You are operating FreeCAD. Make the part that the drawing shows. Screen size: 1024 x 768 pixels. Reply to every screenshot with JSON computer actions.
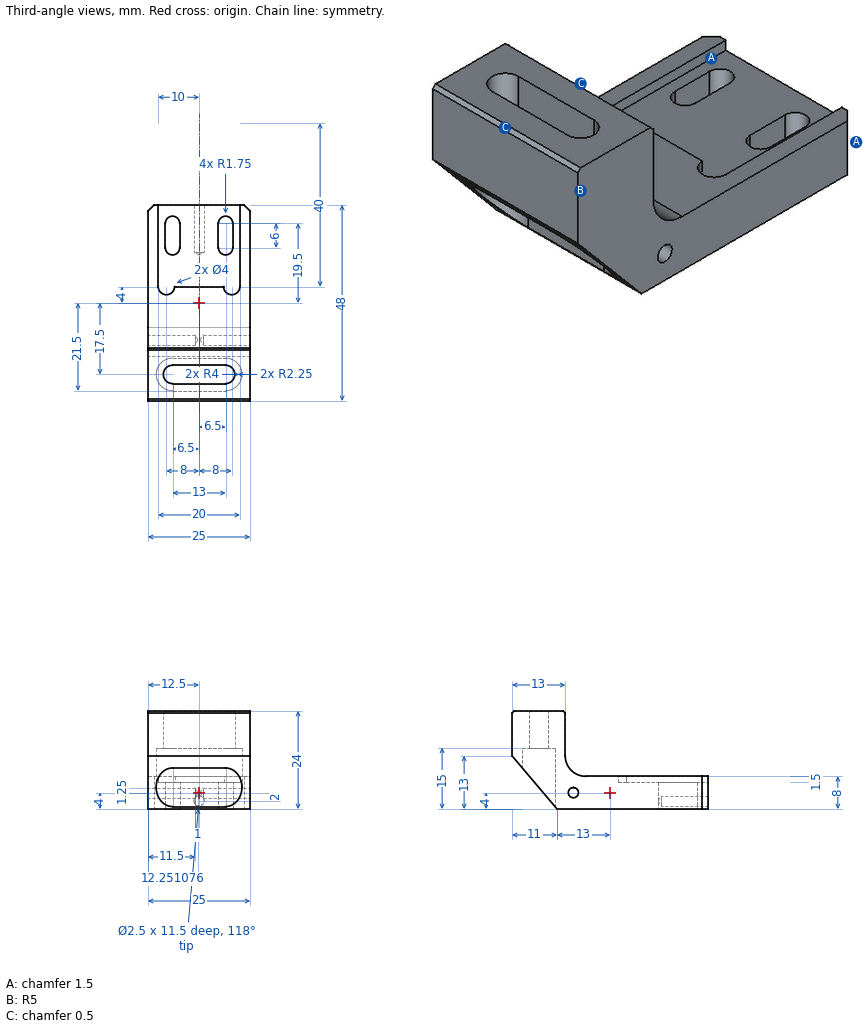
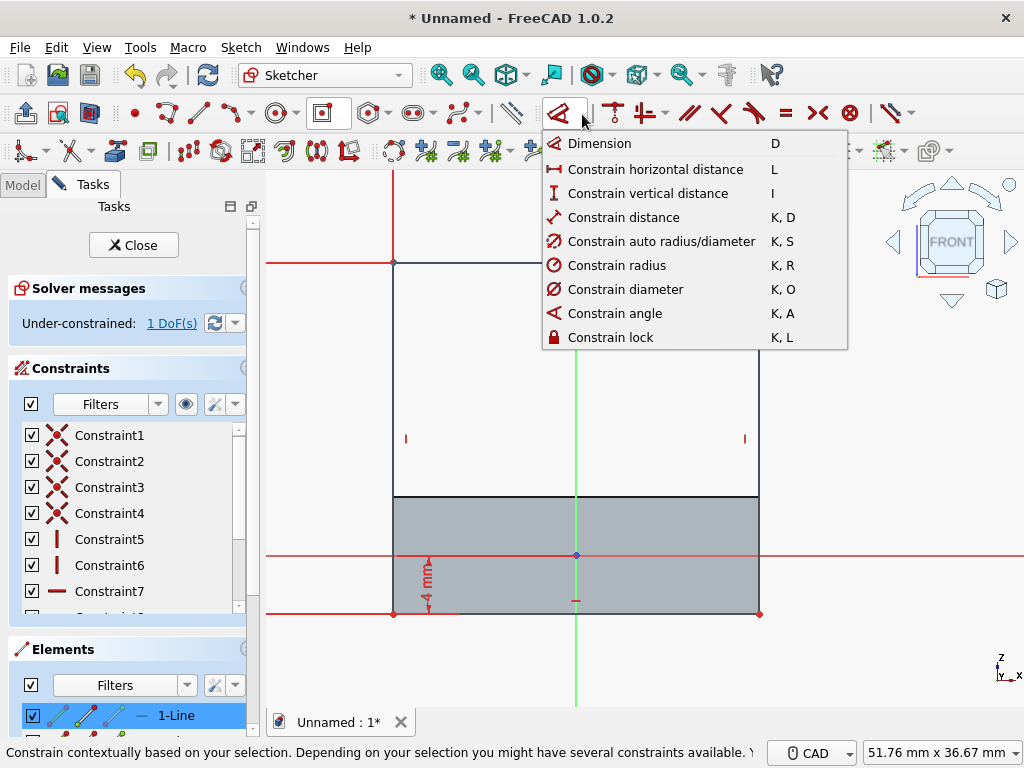
{"action": "left_click", "coordinate": [695, 169]}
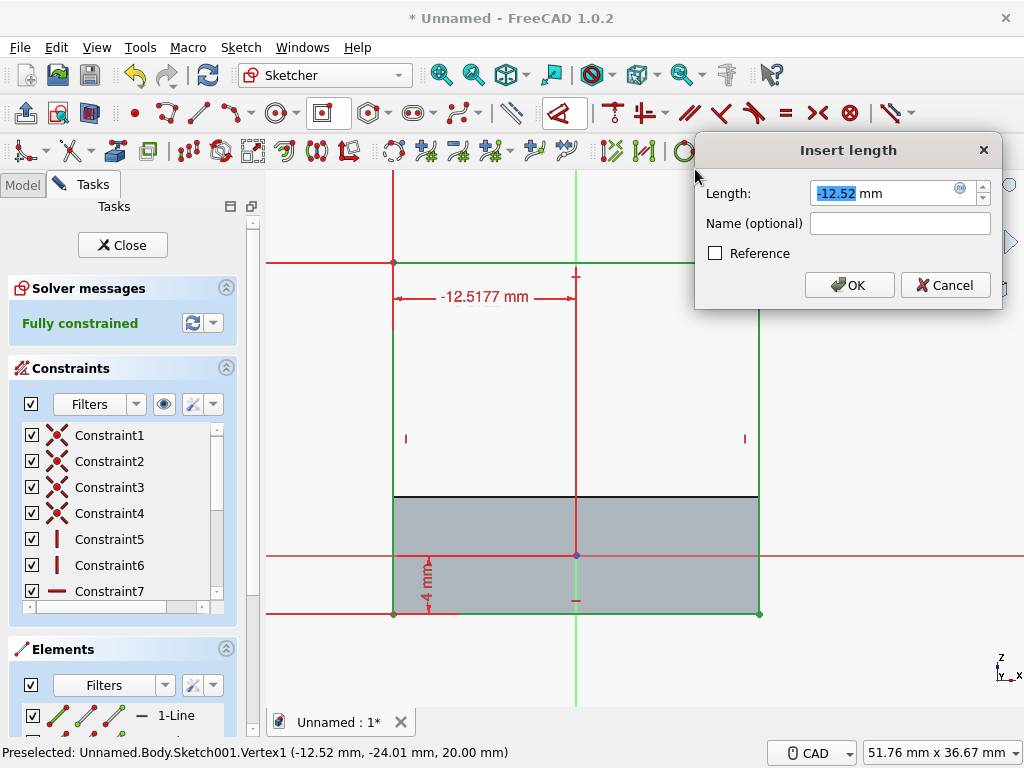
{"action": "type", "text": "-12.5"}
{"action": "key", "text": "Return"}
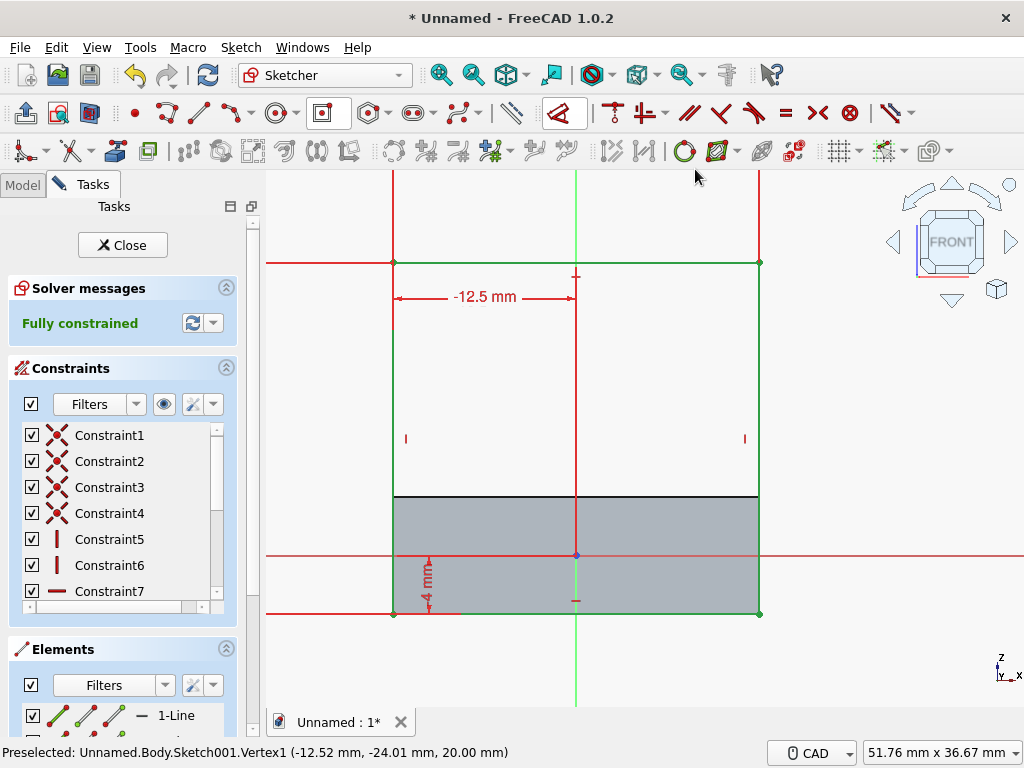
{"action": "left_click", "coordinate": [123, 245]}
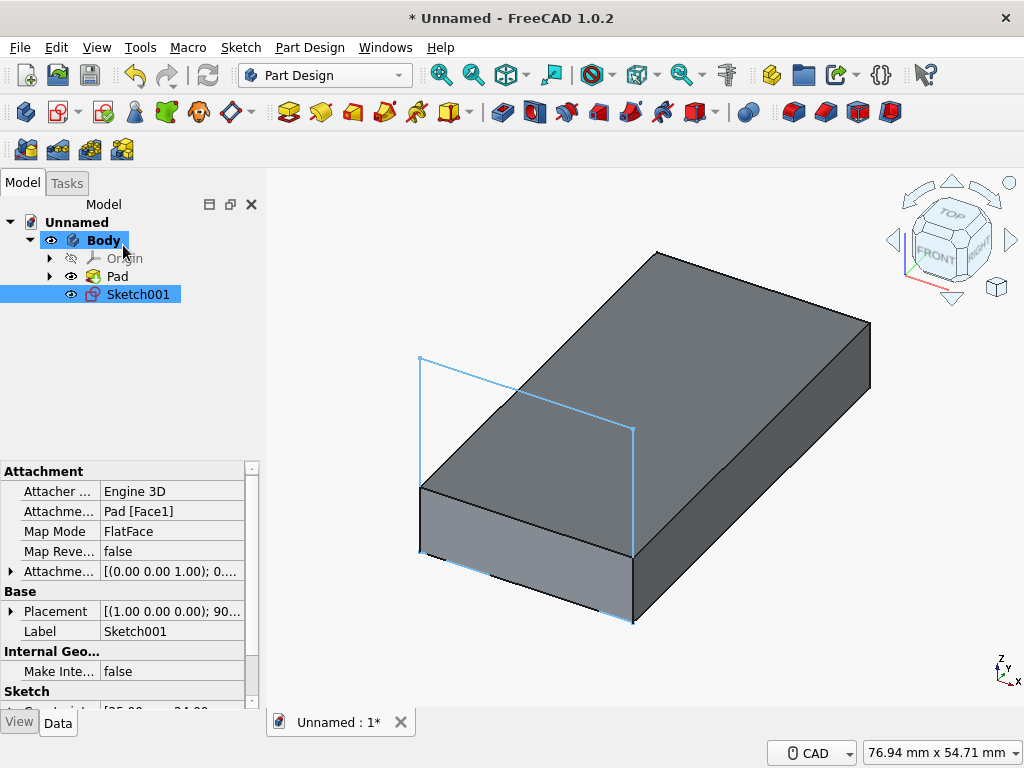
{"action": "left_click", "coordinate": [290, 112]}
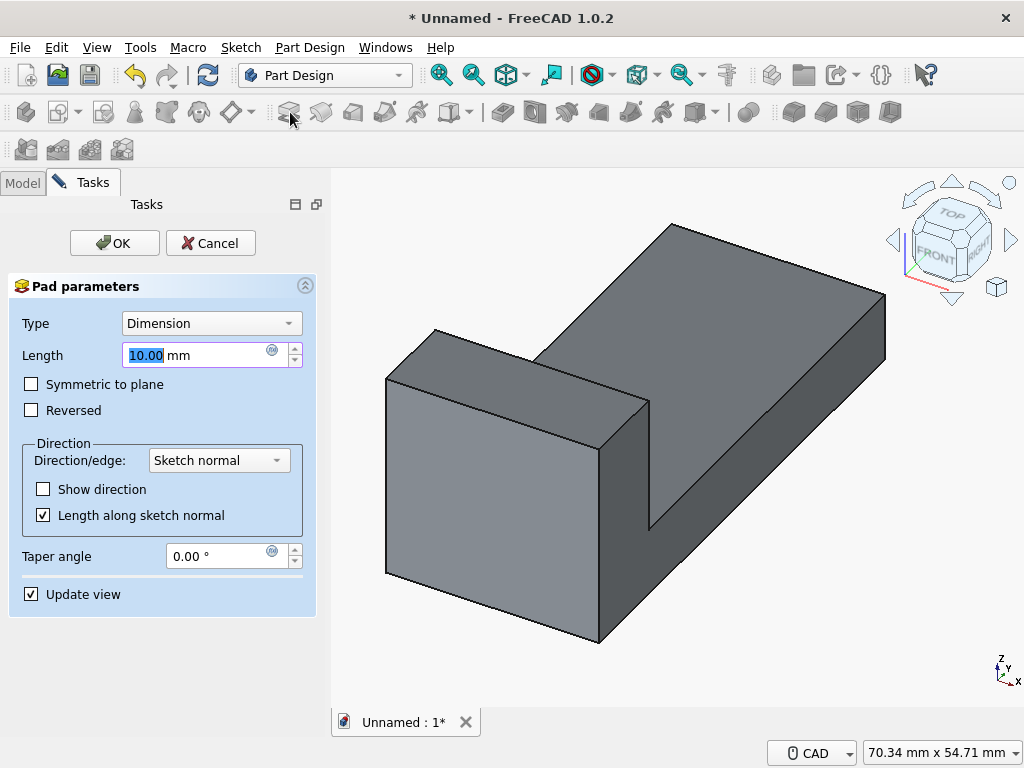
{"action": "type", "text": "13"}
{"action": "key", "text": "Tab"}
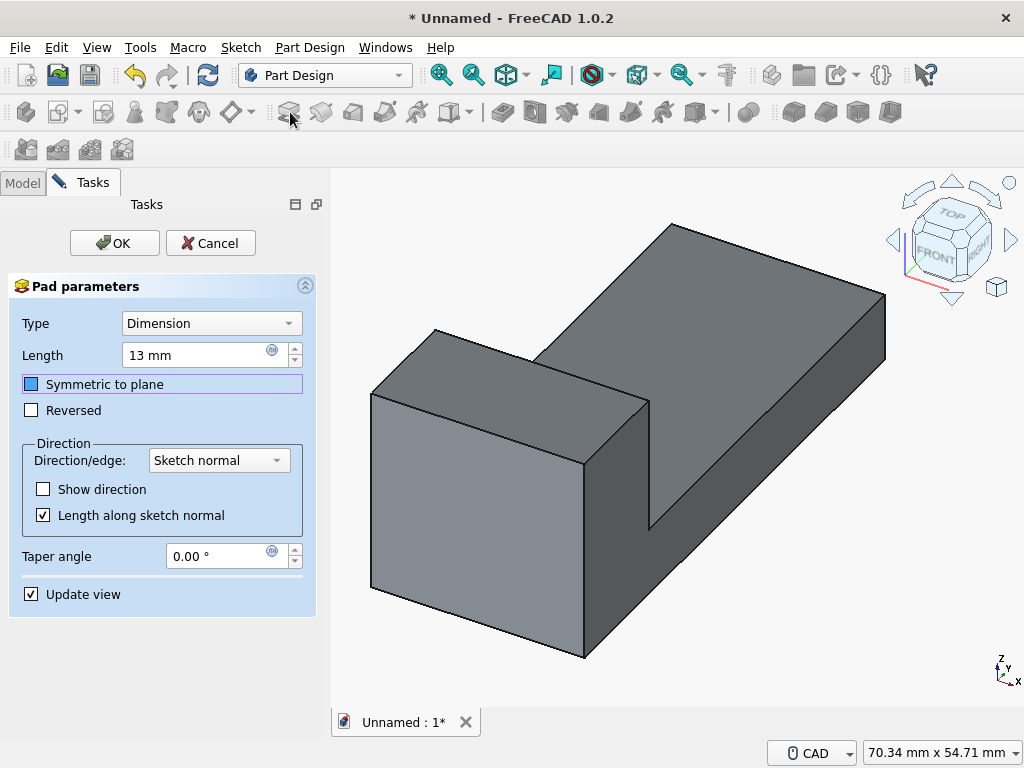
{"action": "left_click", "coordinate": [30, 410]}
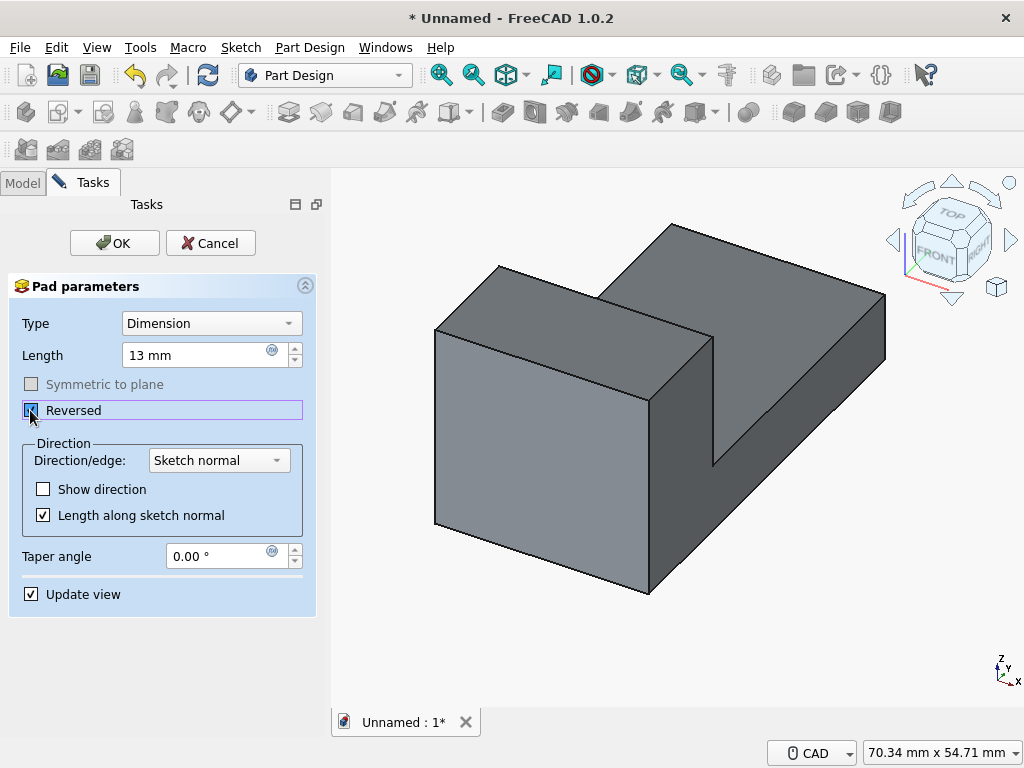
{"action": "left_click", "coordinate": [115, 243]}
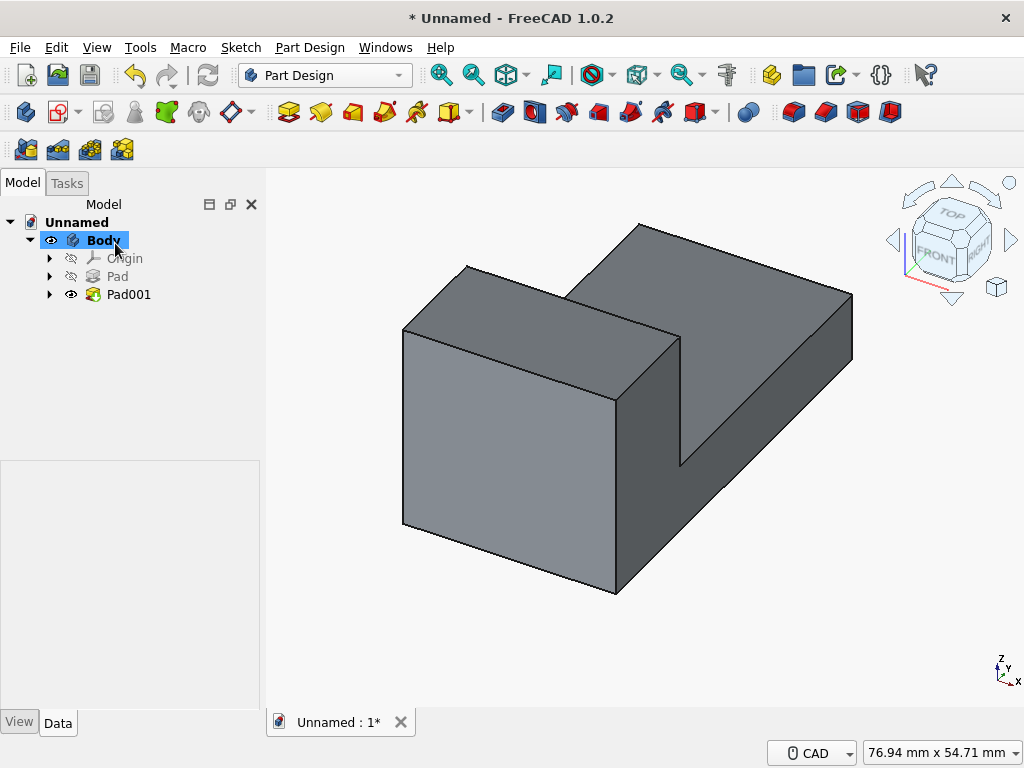
{"action": "left_click", "coordinate": [442, 76]}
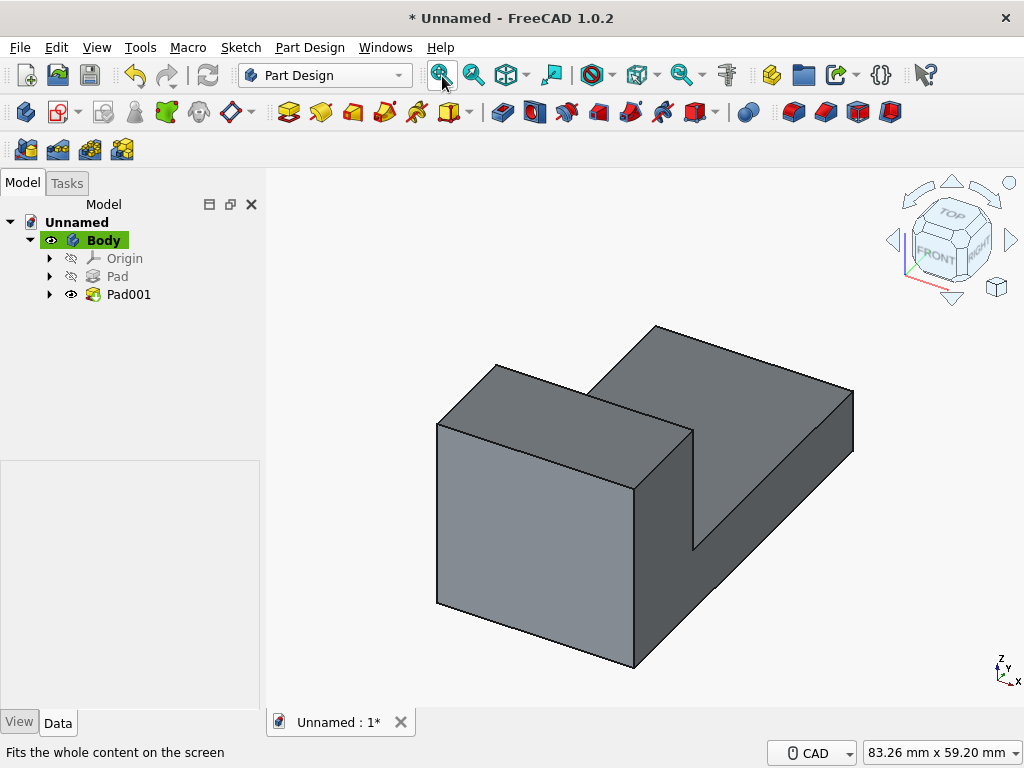
{"action": "left_click", "coordinate": [697, 414]}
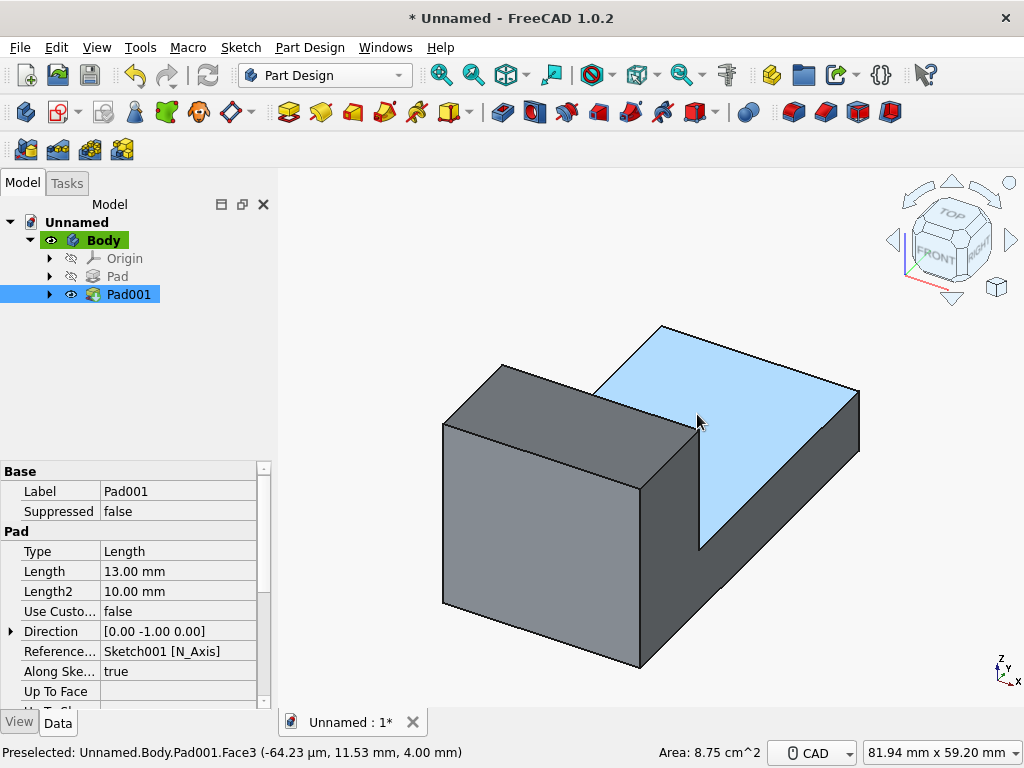
{"action": "left_click", "coordinate": [58, 112]}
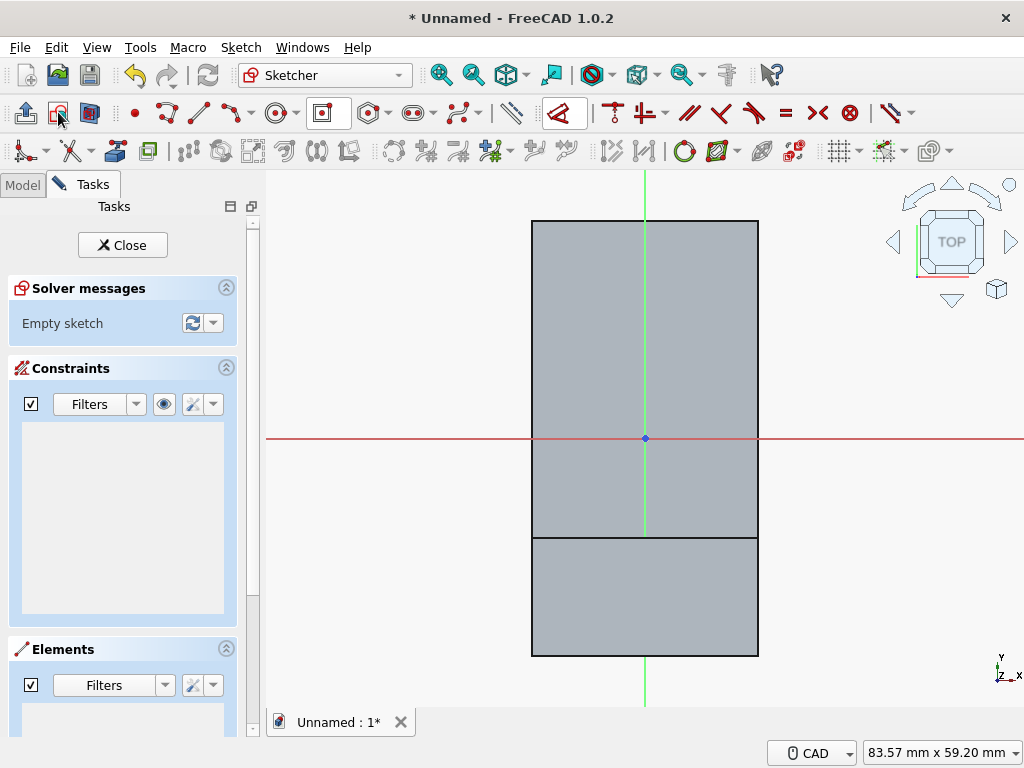
{"action": "scroll", "coordinate": [437, 679], "scroll_direction": "down", "scroll_amount": 2}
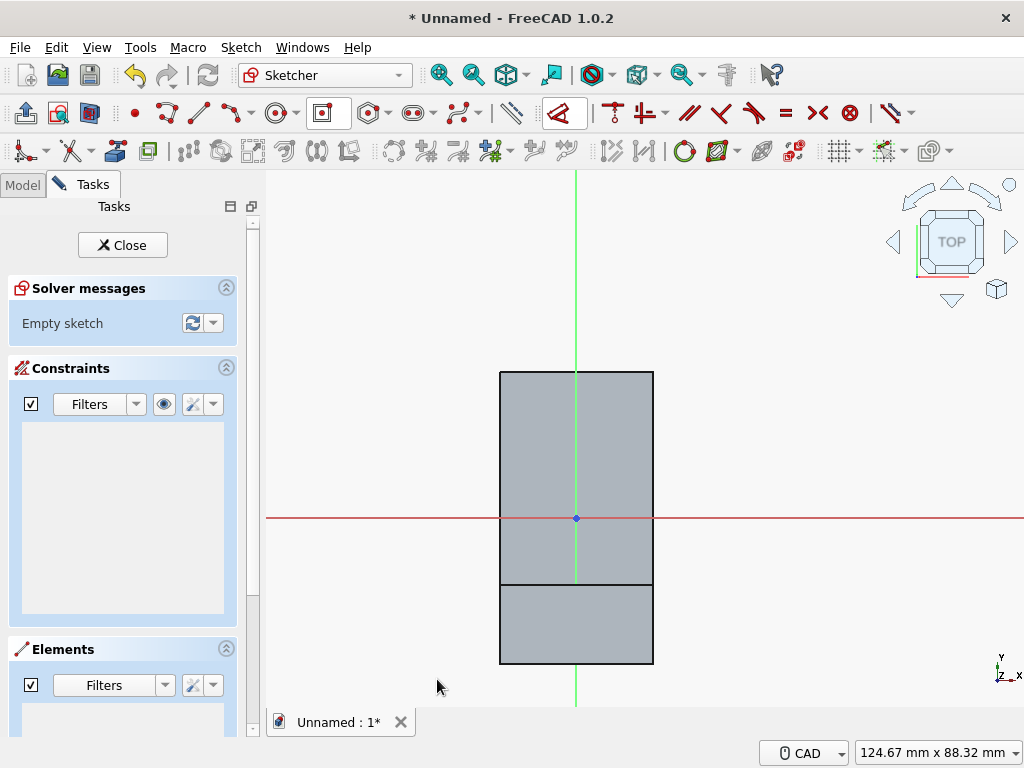
{"action": "key", "text": "g r"}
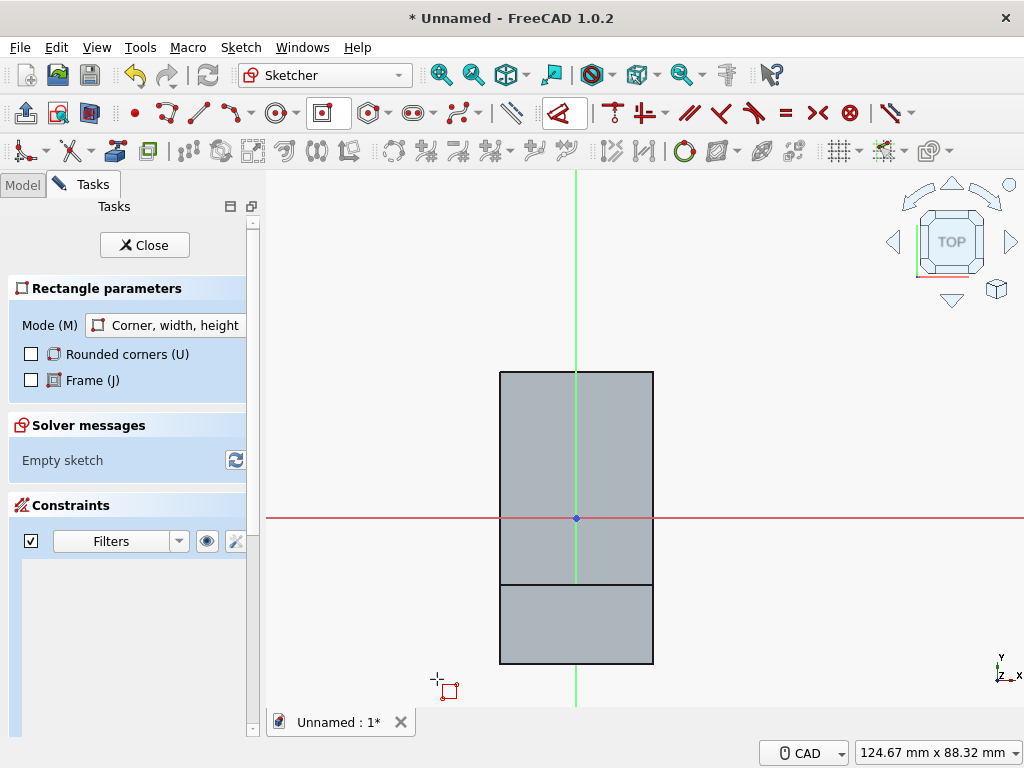
{"action": "left_click", "coordinate": [516, 251]}
{"action": "mouse_move", "coordinate": [637, 494]}